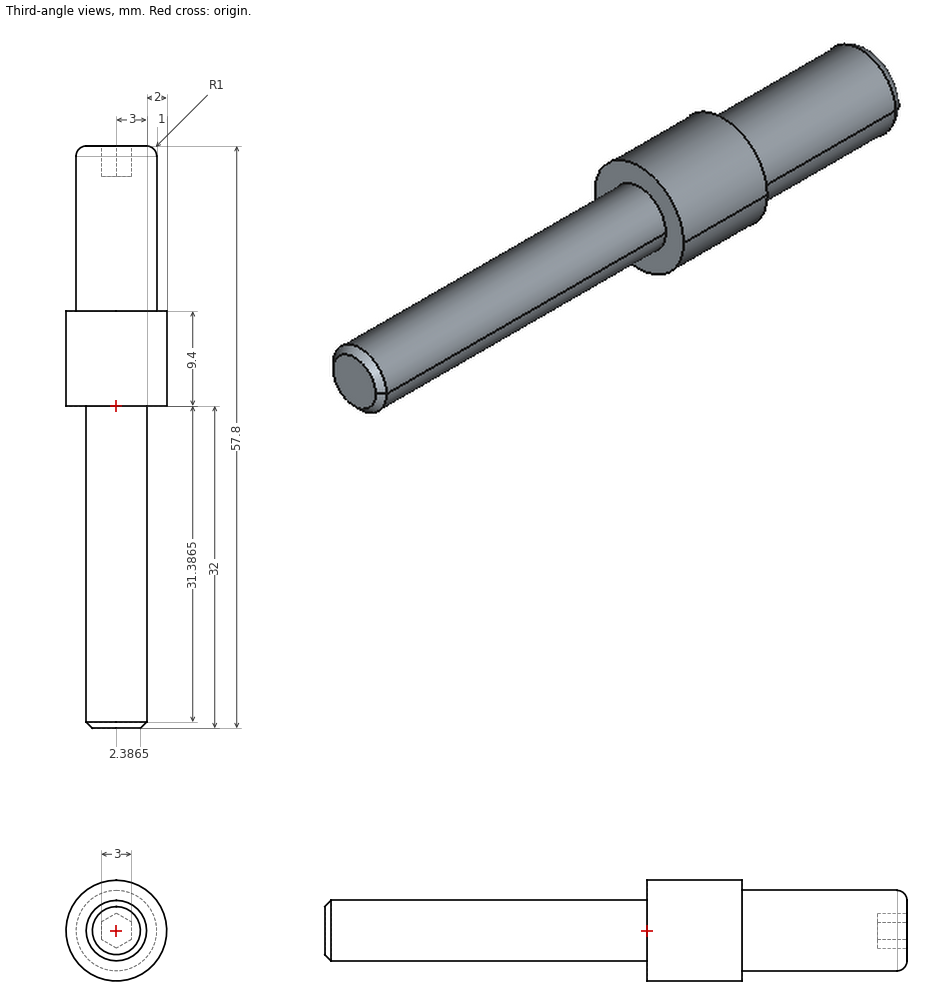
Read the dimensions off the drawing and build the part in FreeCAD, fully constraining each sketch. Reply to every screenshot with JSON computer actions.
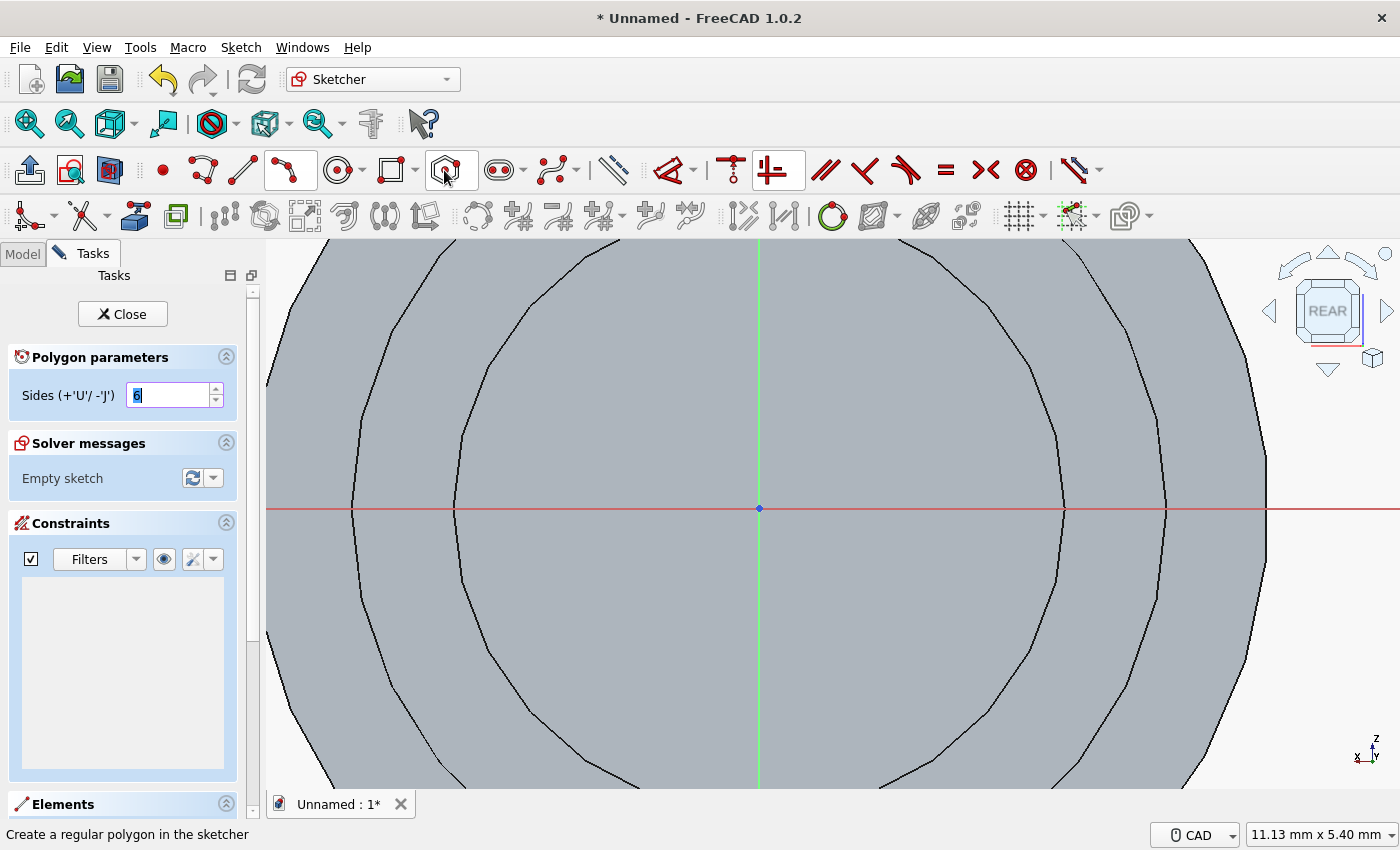
{"action": "left_click", "coordinate": [759, 509]}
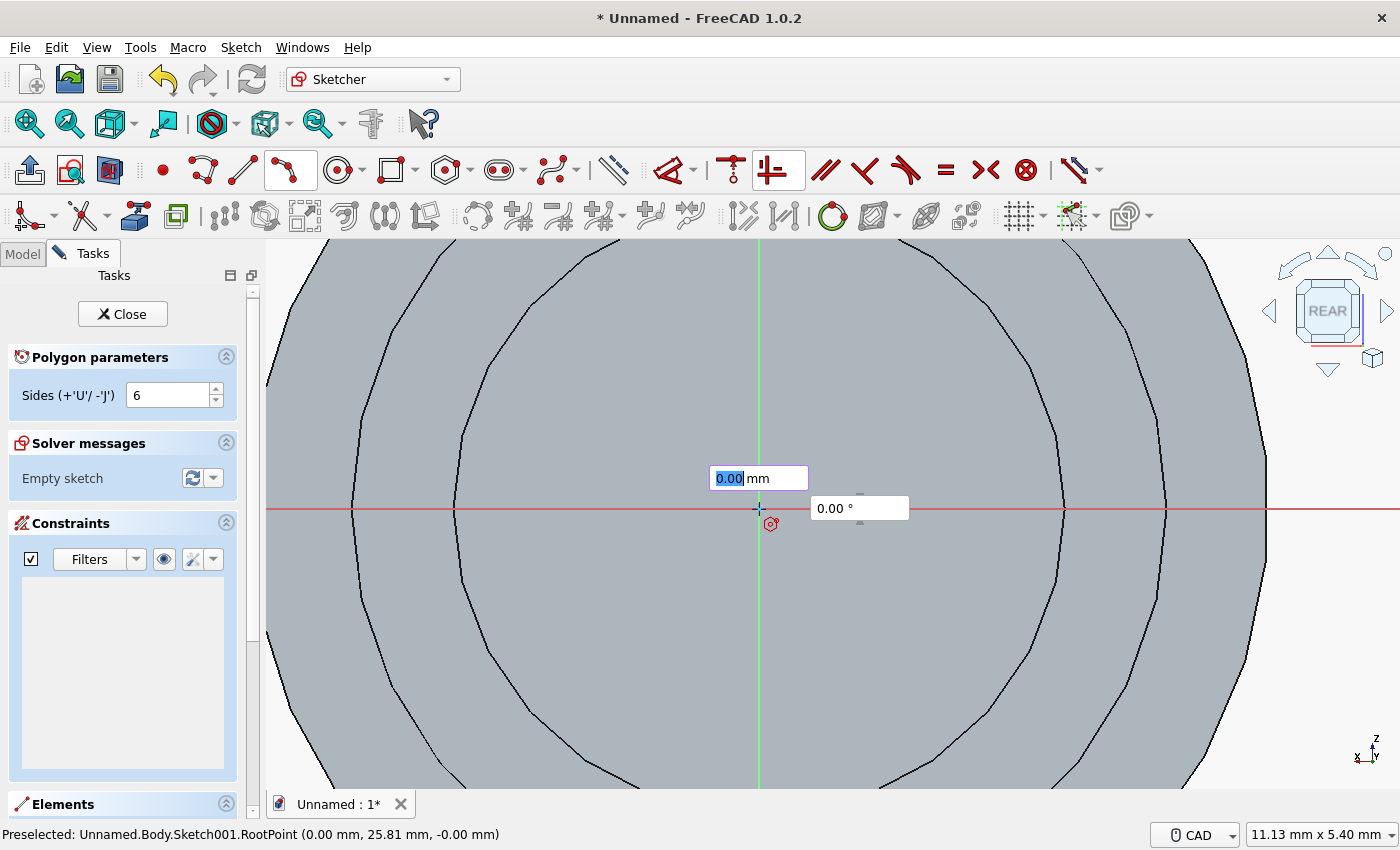
{"action": "left_click", "coordinate": [759, 332]}
{"action": "key", "text": "Escape"}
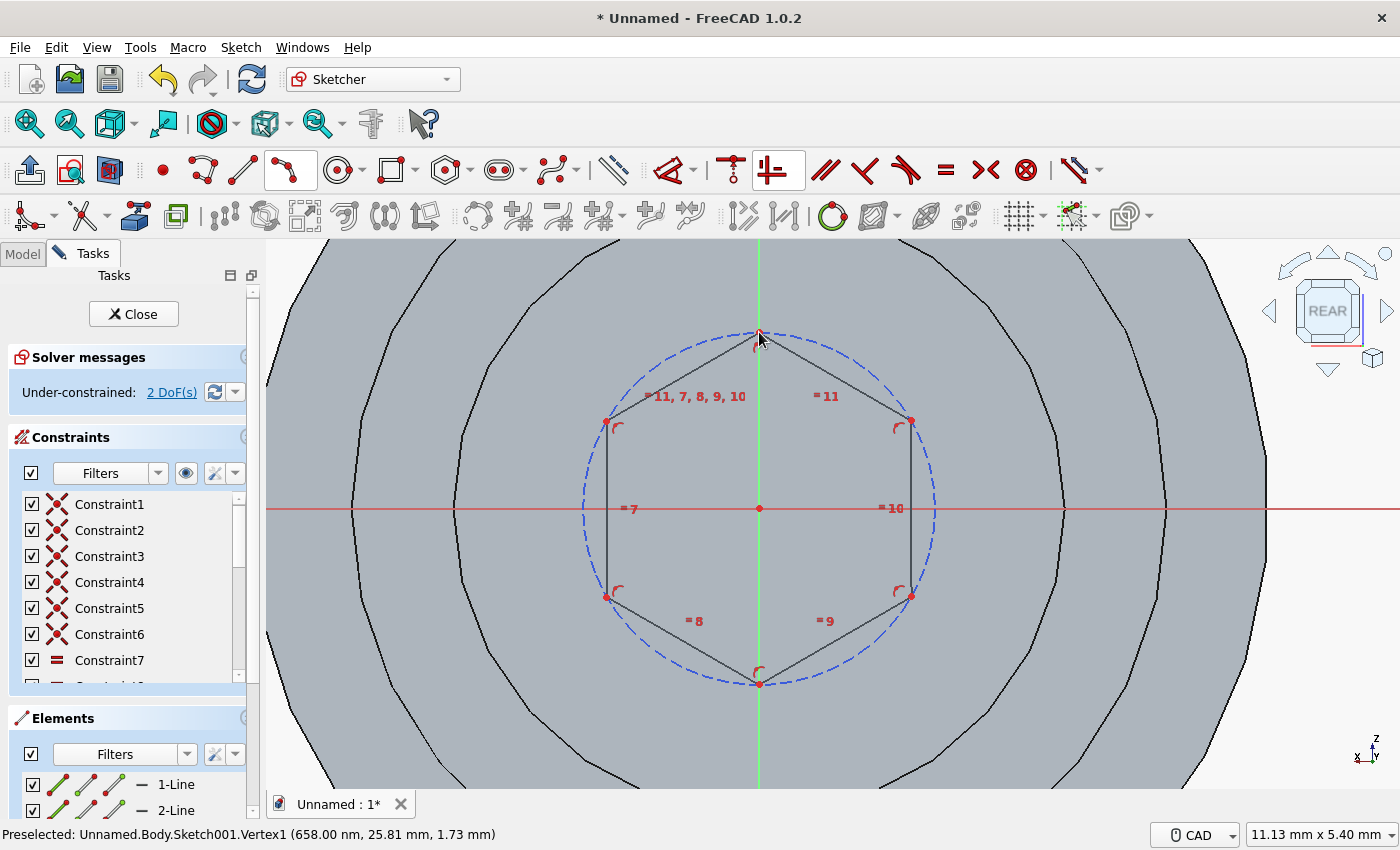
{"action": "left_click", "coordinate": [607, 474]}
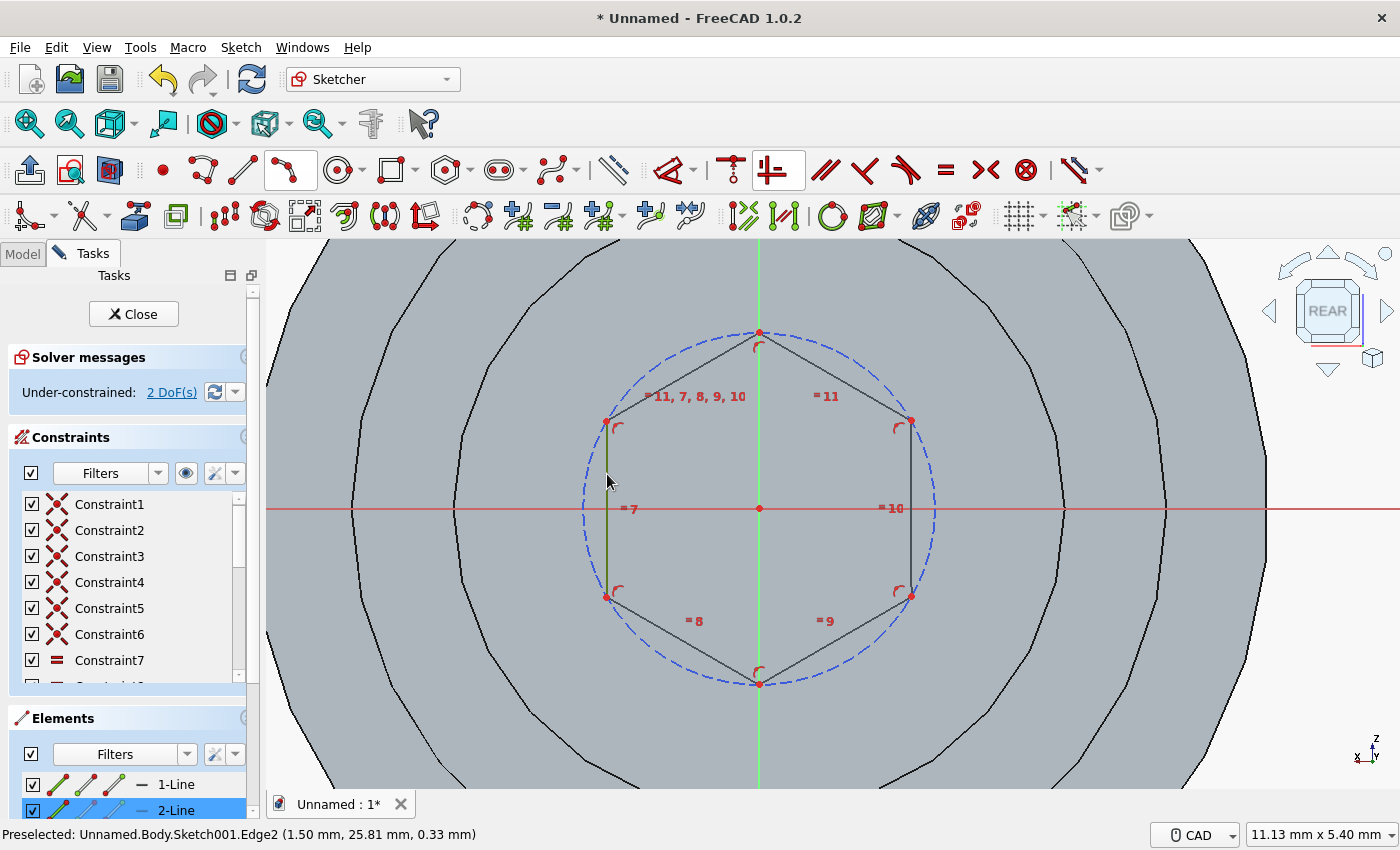
{"action": "left_click", "coordinate": [800, 170]}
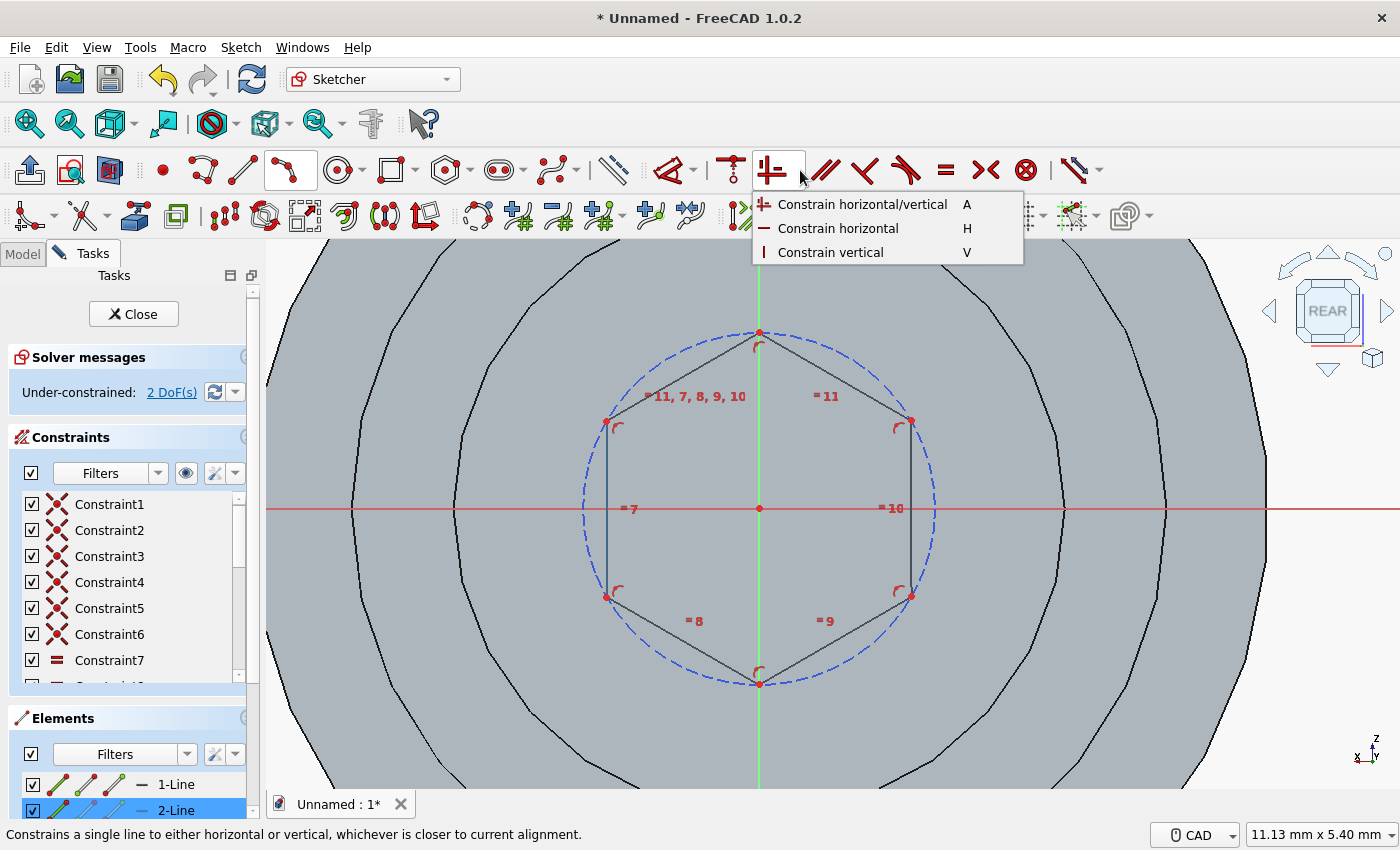
{"action": "left_click", "coordinate": [888, 252]}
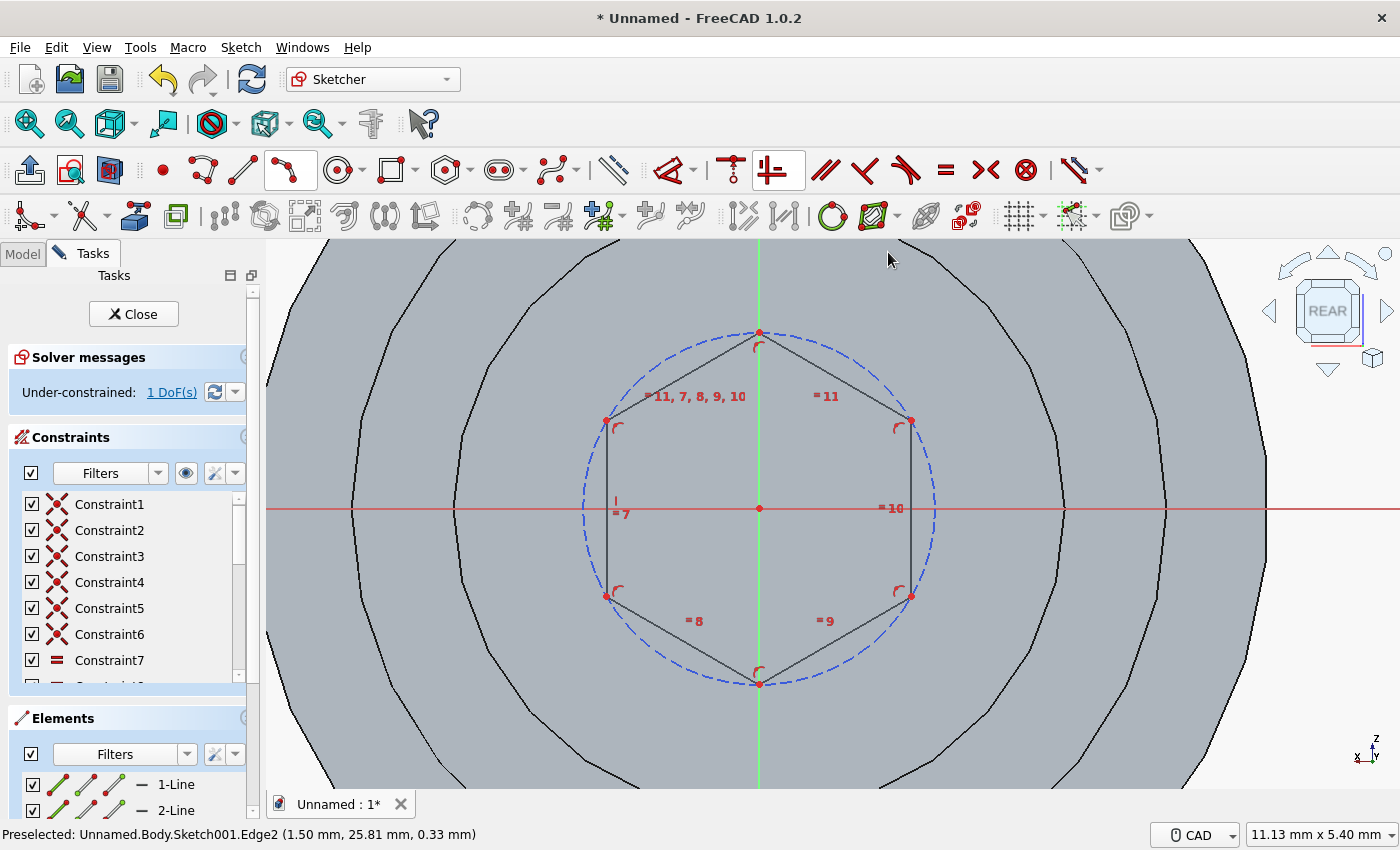
{"action": "left_click", "coordinate": [668, 170]}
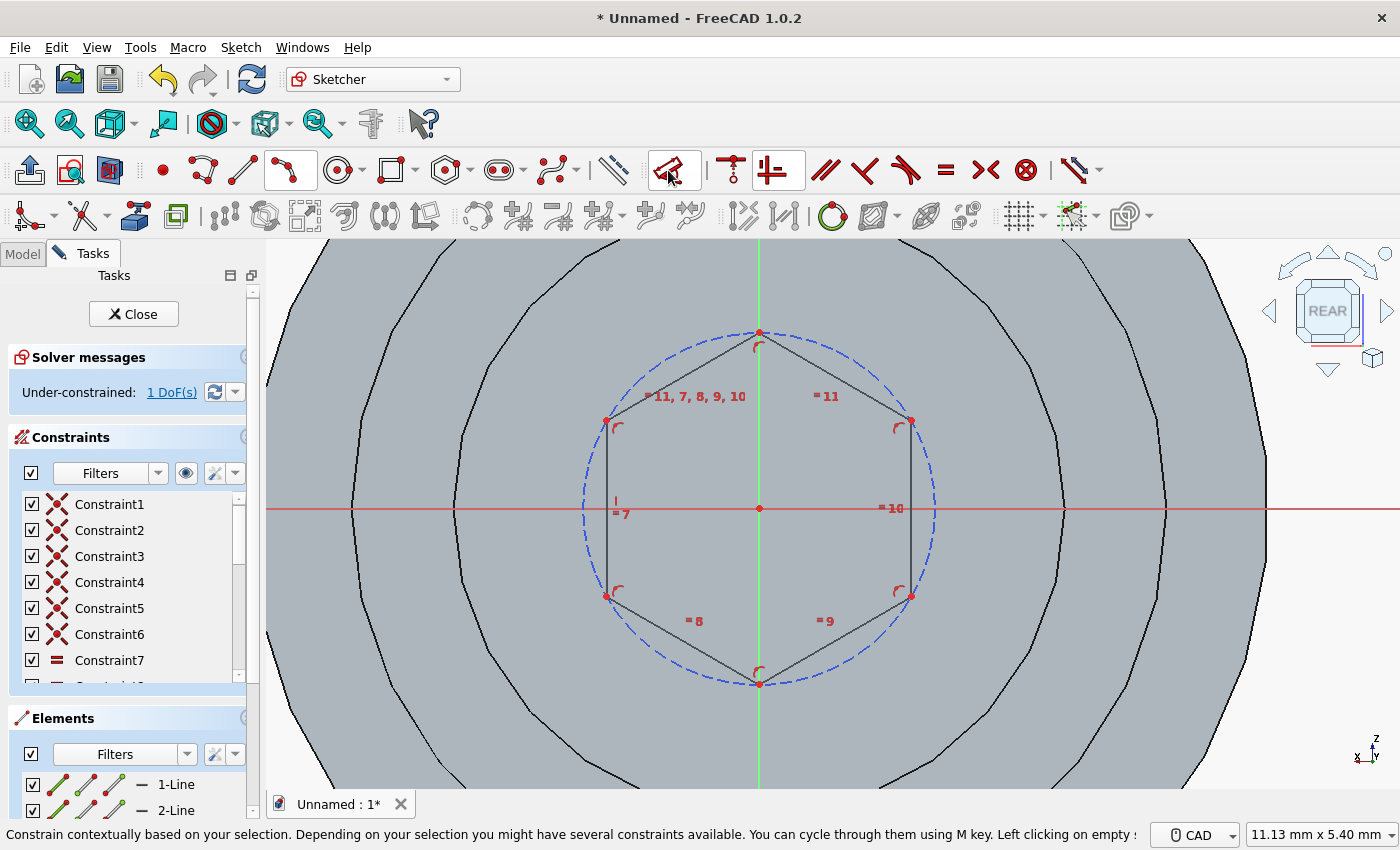
{"action": "left_click", "coordinate": [607, 421]}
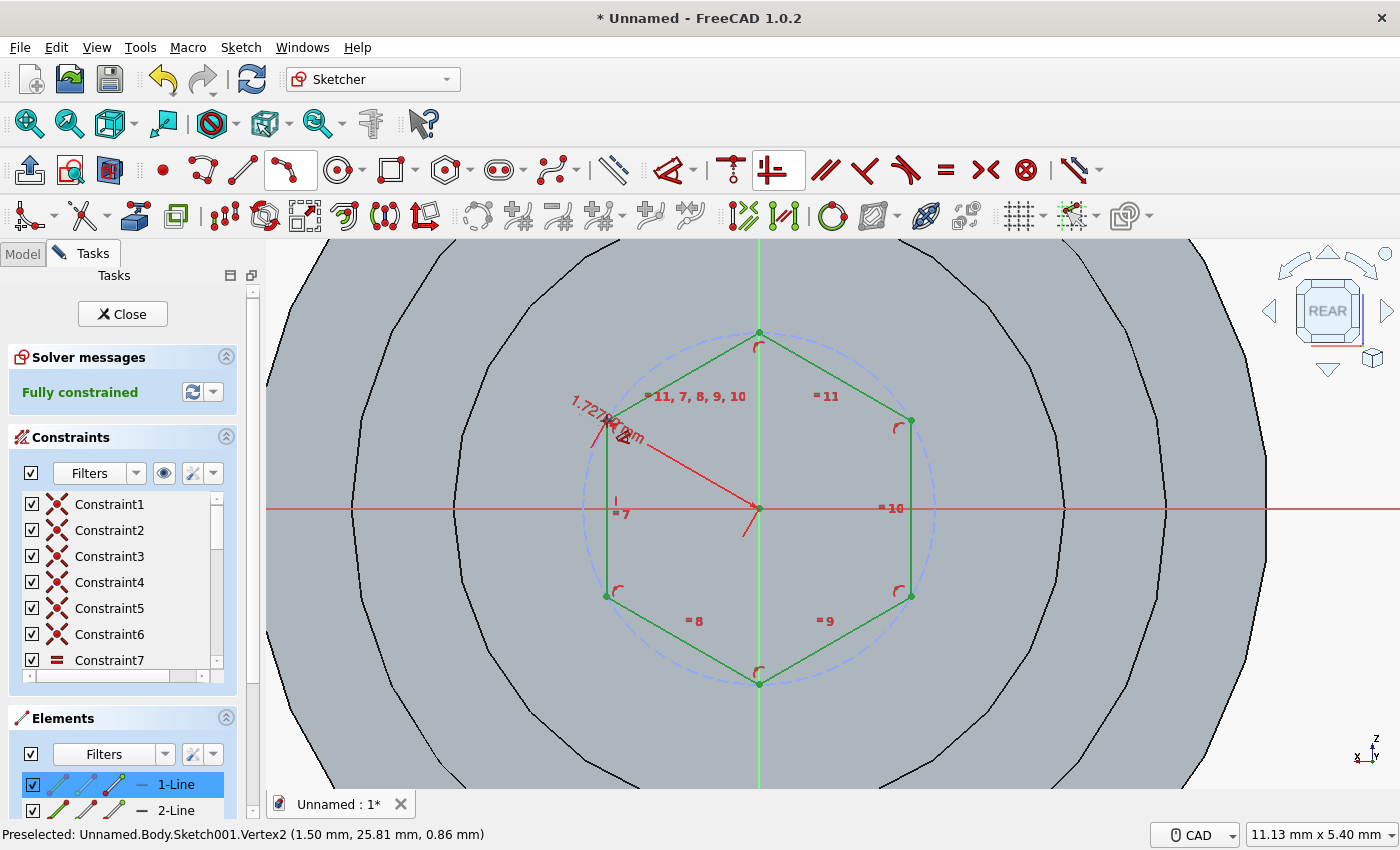
{"action": "left_click", "coordinate": [911, 597]}
{"action": "left_click", "coordinate": [652, 679]}